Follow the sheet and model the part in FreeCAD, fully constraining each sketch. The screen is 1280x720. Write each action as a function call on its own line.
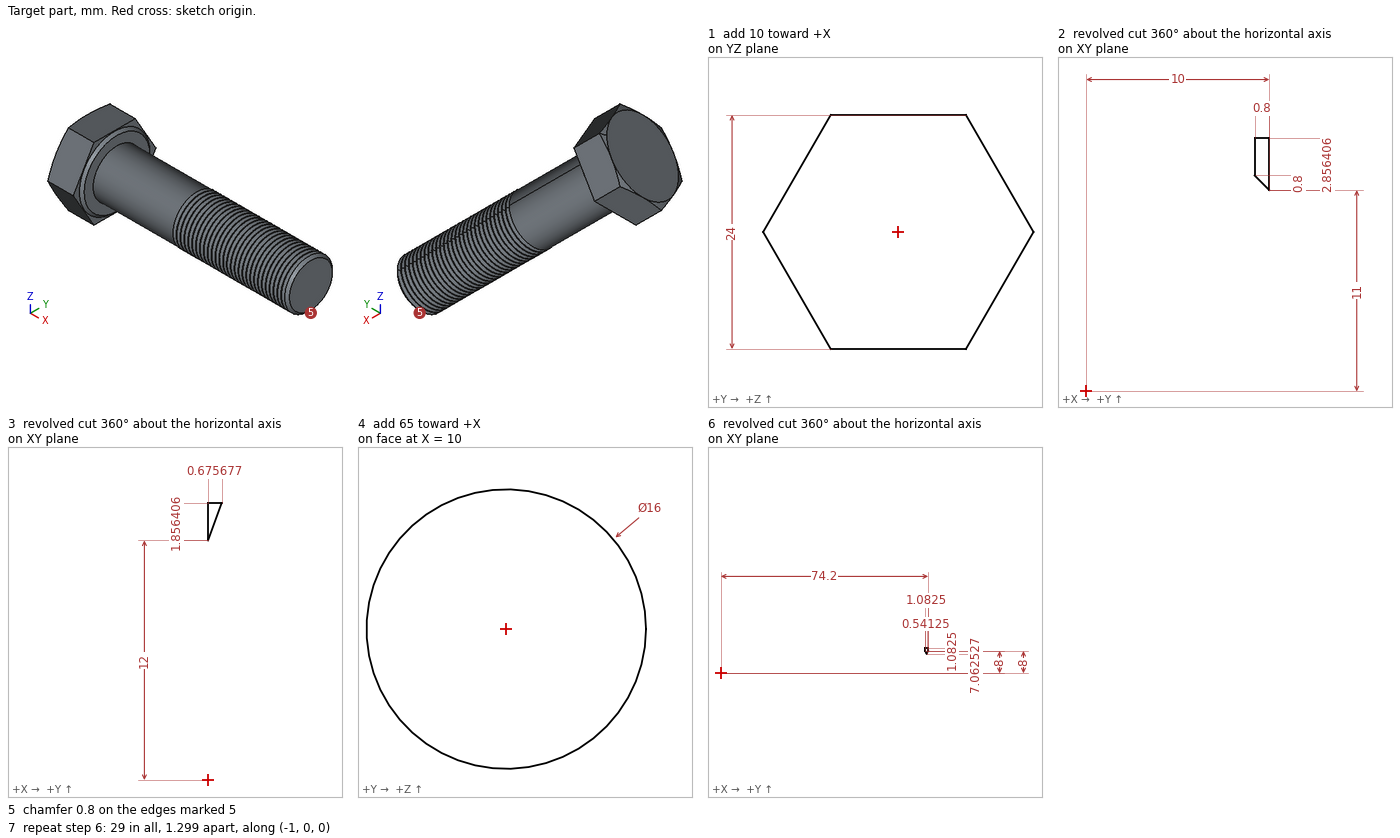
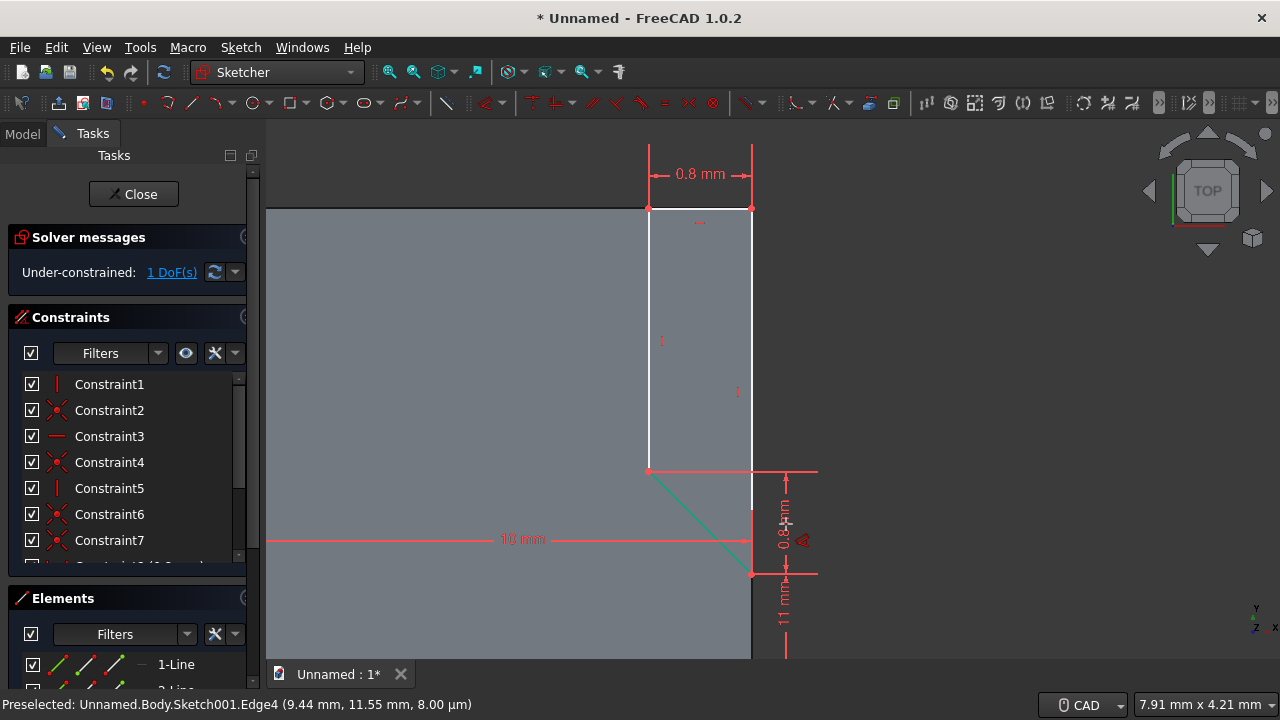
click(752, 465)
click(786, 392)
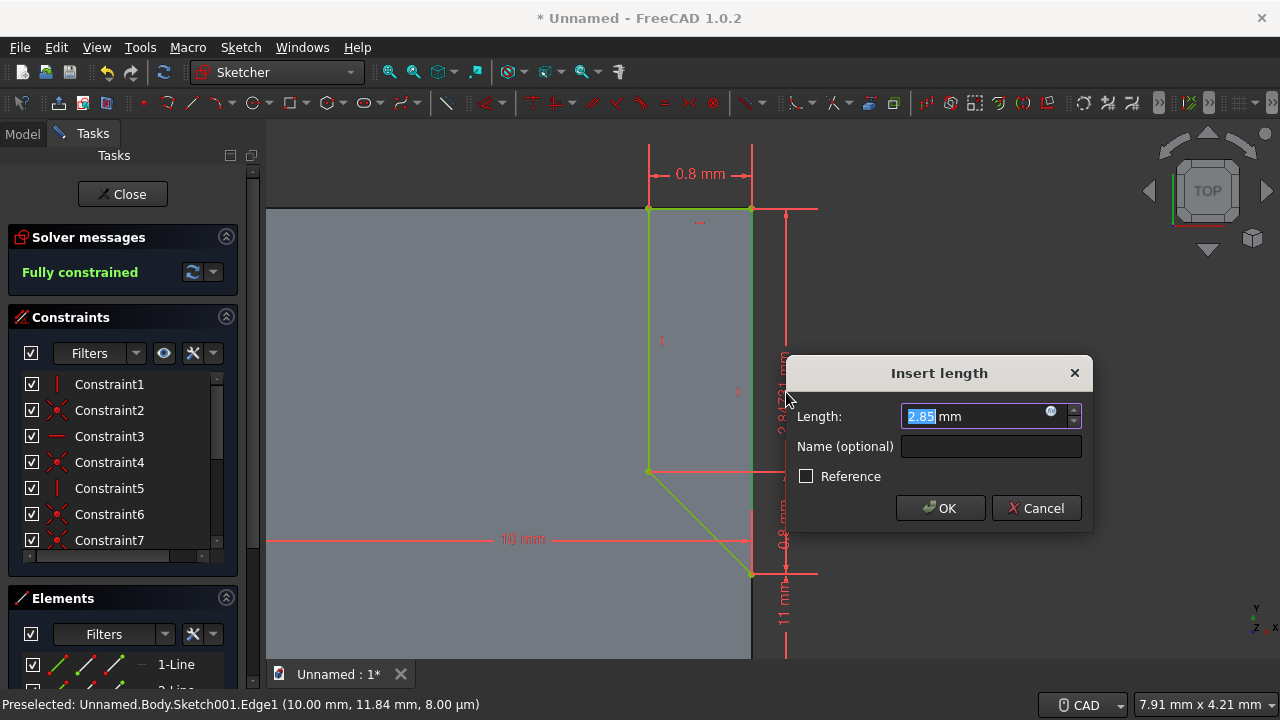
text(2.856406)
key(Return)
key(Escape)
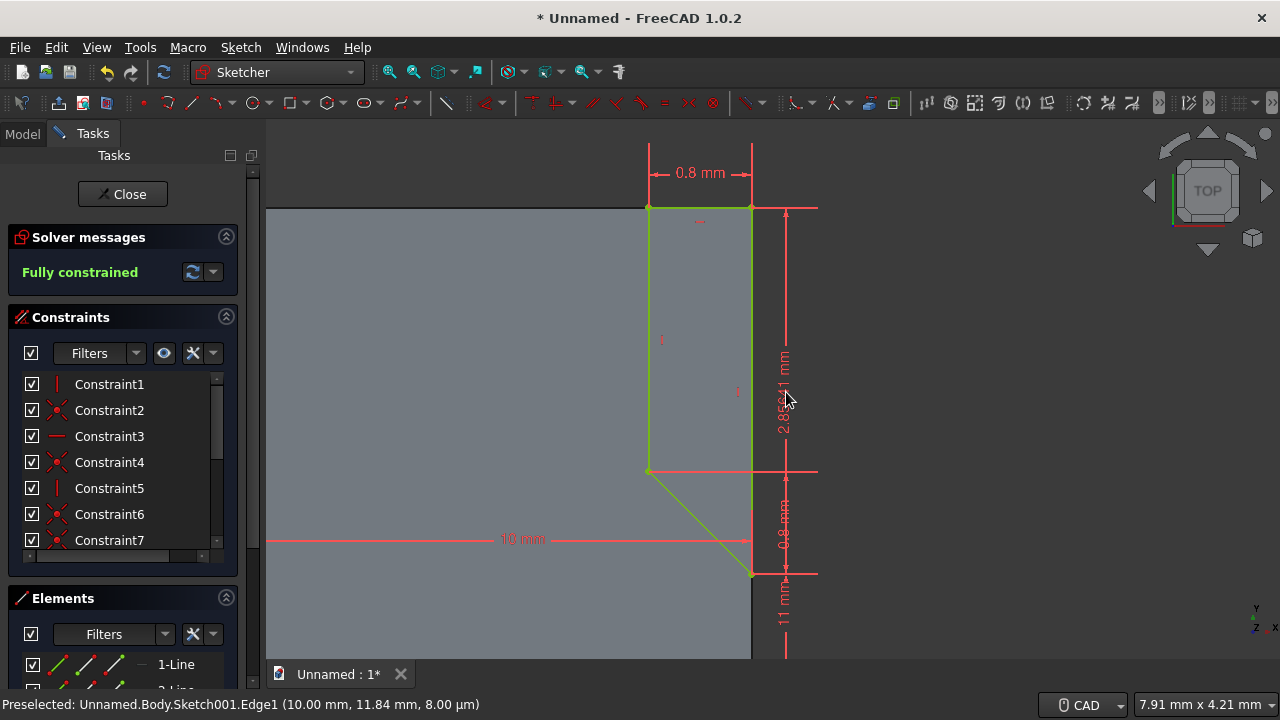
click(123, 194)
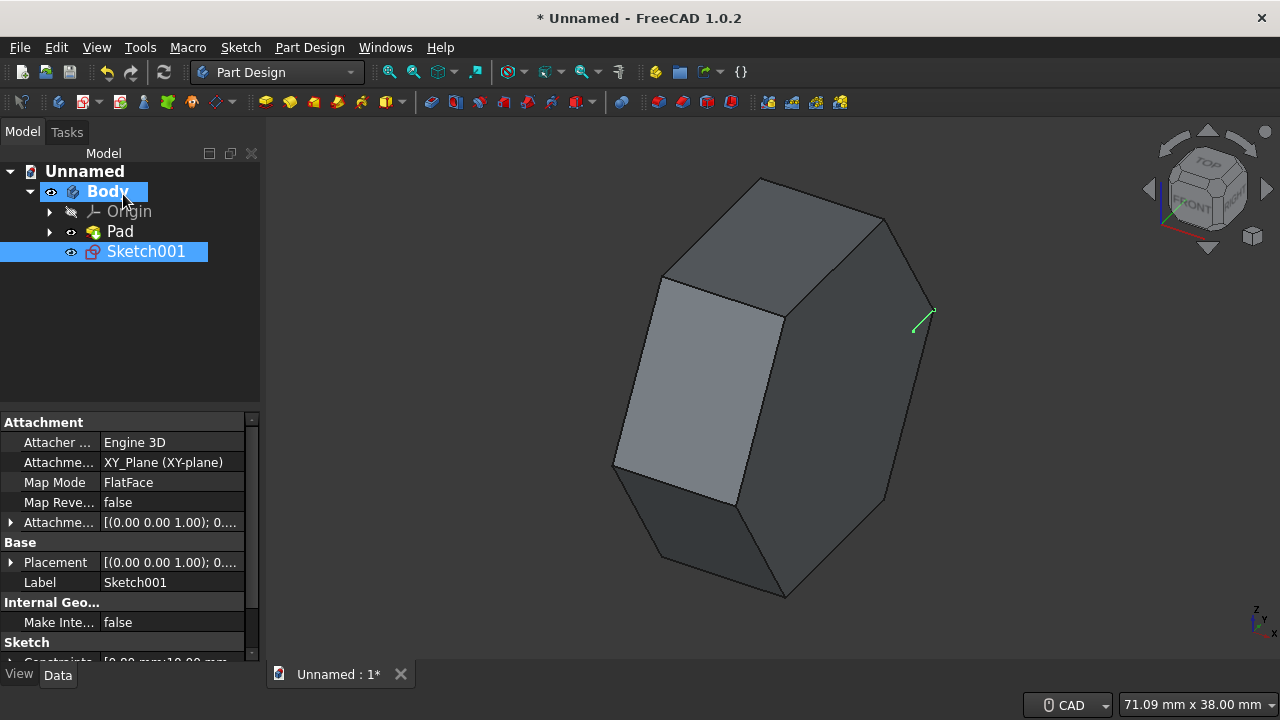
click(480, 102)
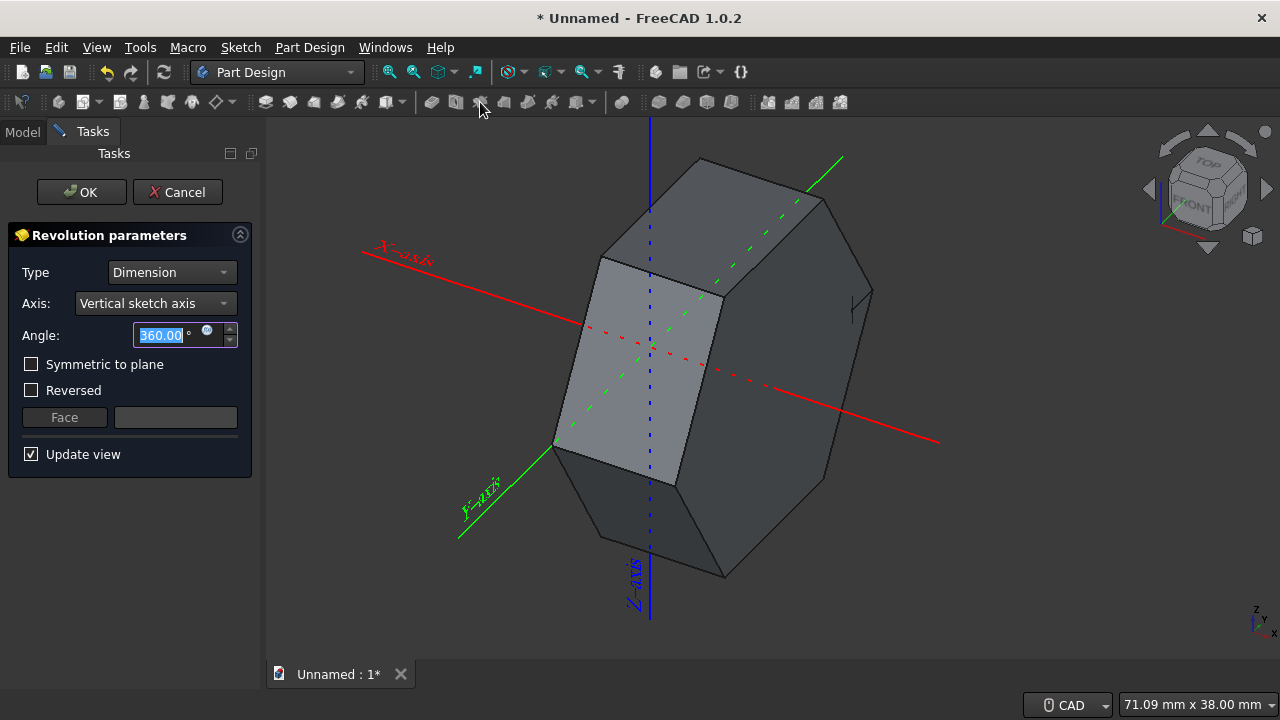
click(156, 304)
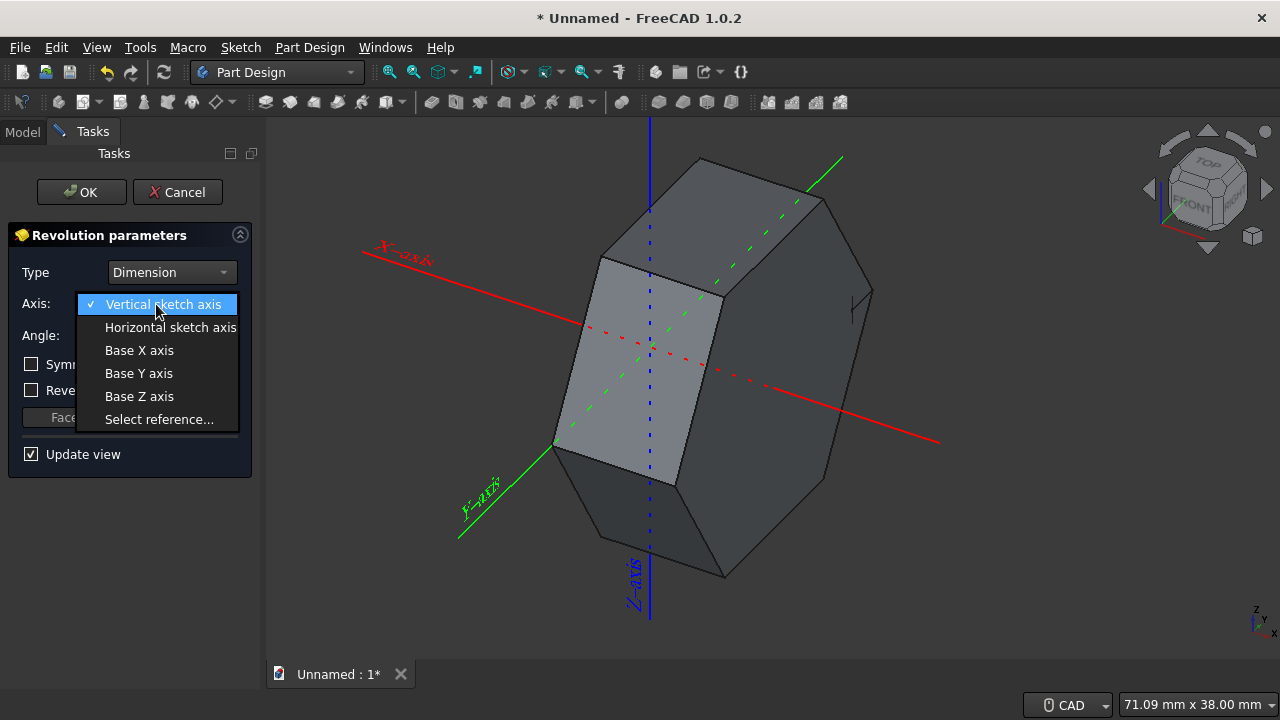
click(156, 328)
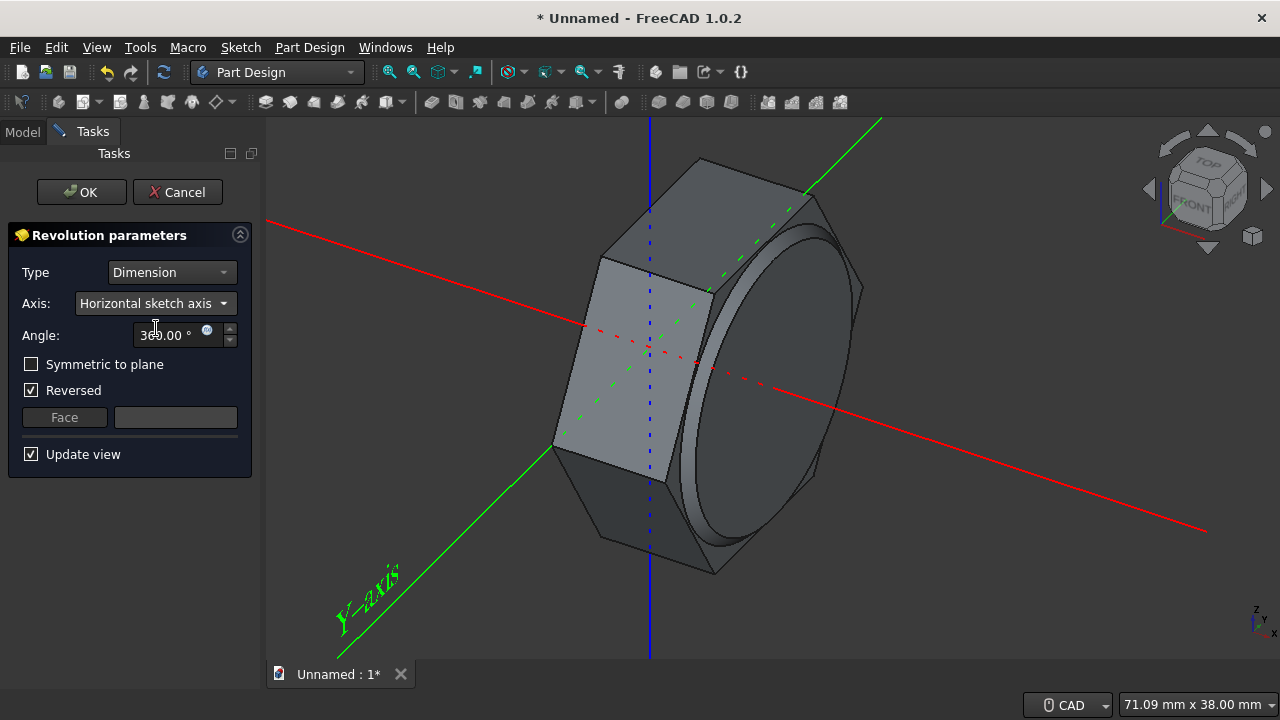
click(82, 192)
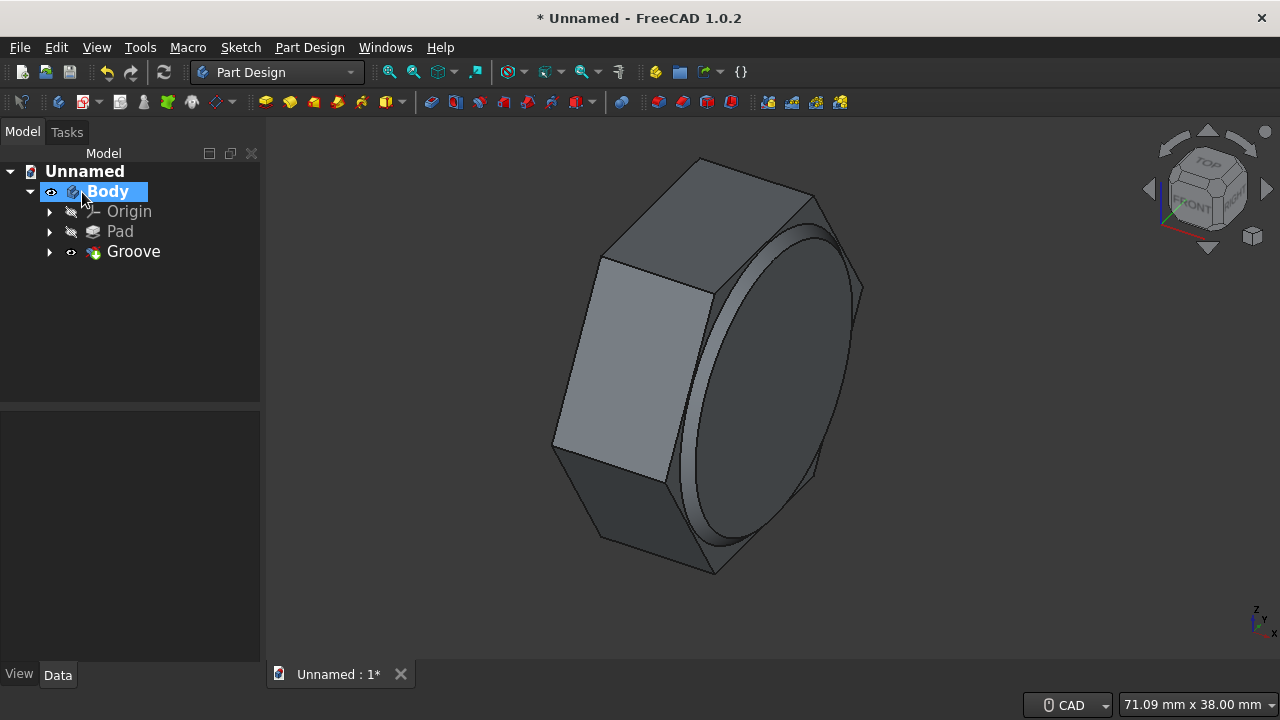
click(390, 72)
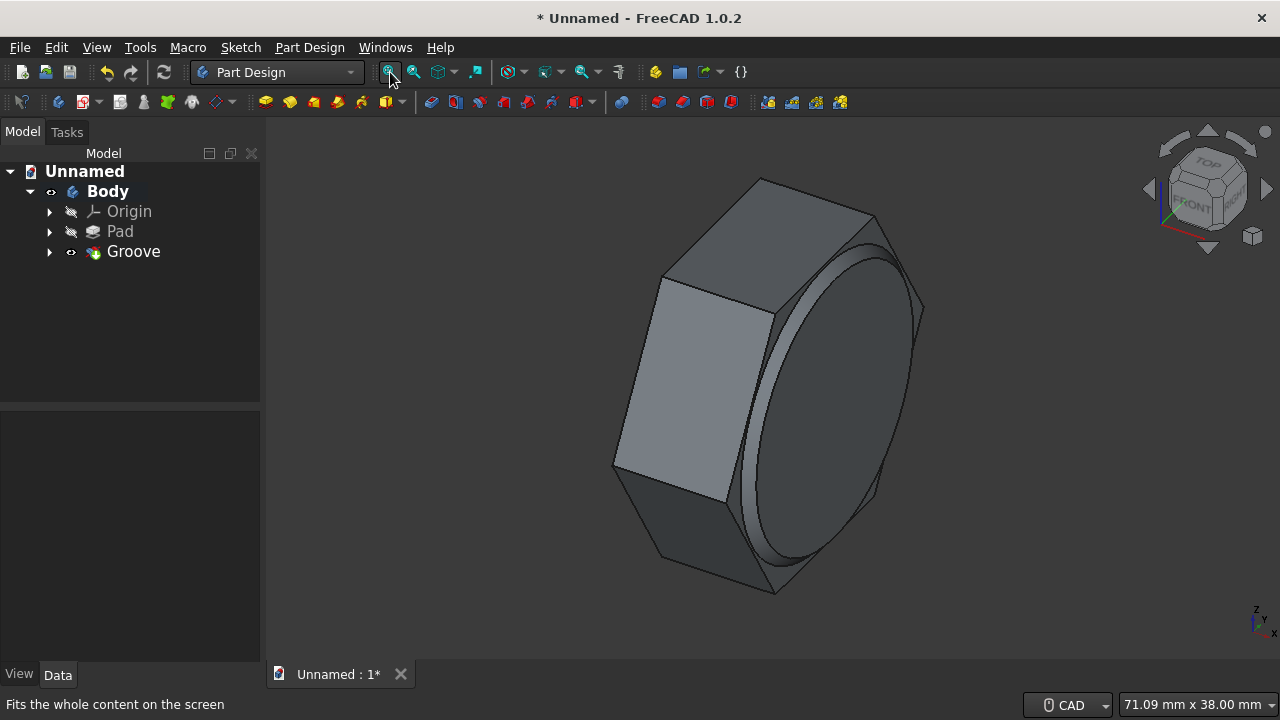
click(84, 102)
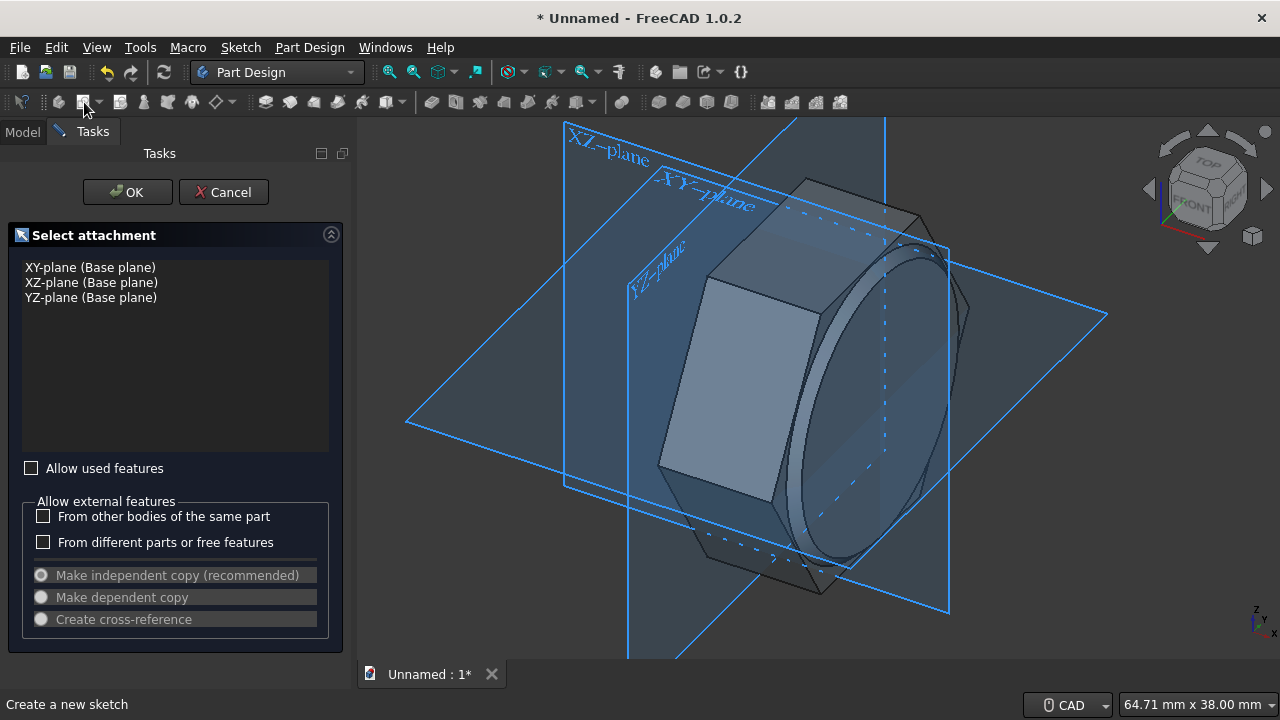
click(82, 268)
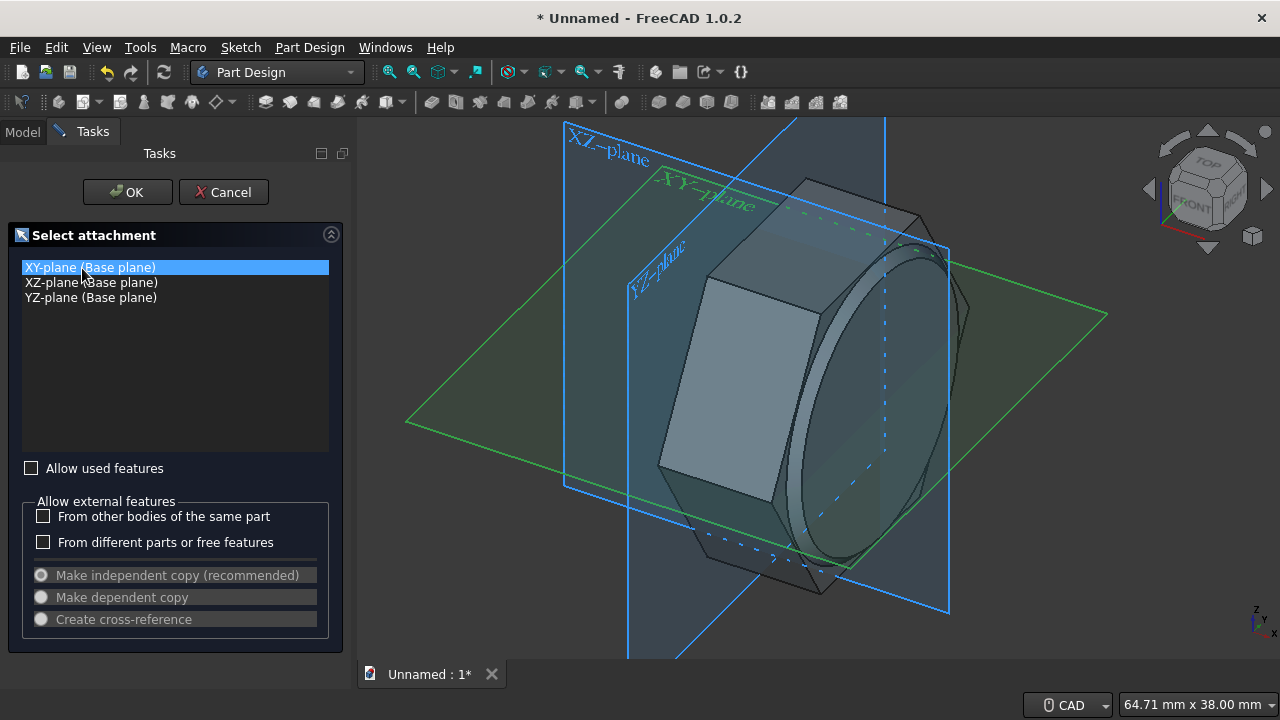
click(128, 192)